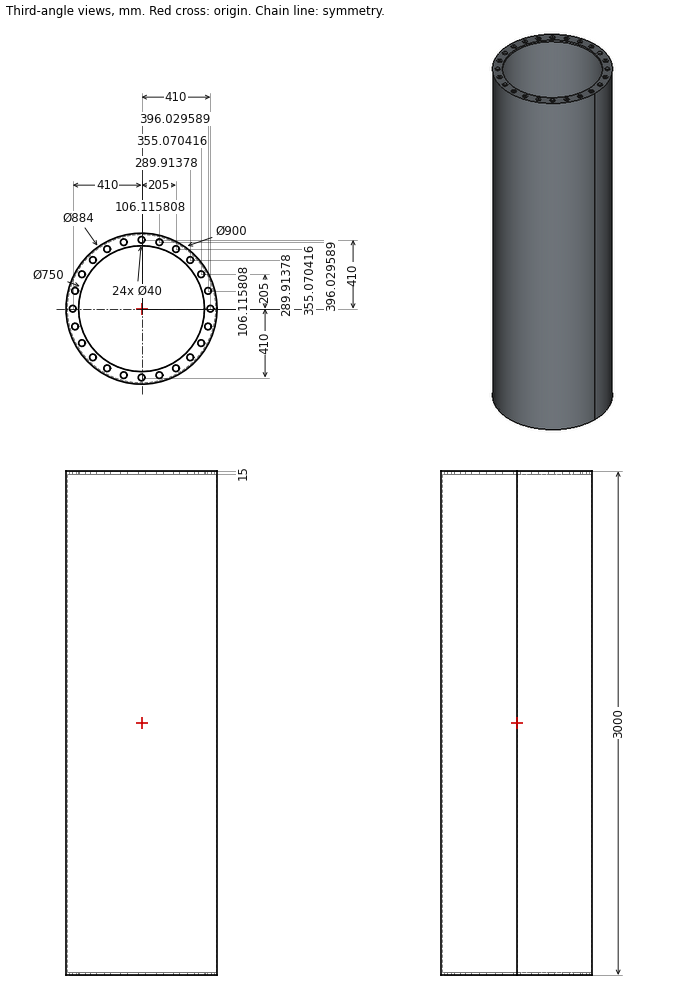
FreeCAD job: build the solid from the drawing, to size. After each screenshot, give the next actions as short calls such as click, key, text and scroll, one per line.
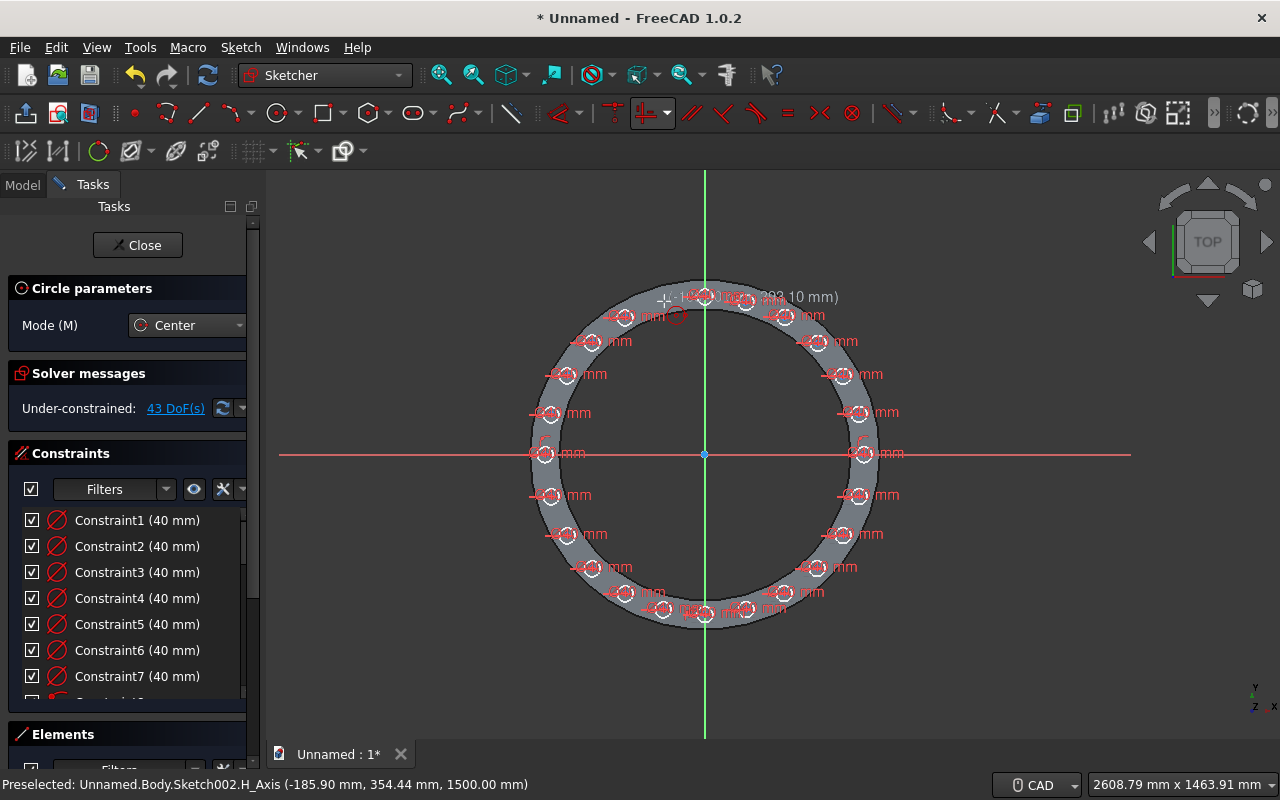
click(664, 301)
move(669, 295)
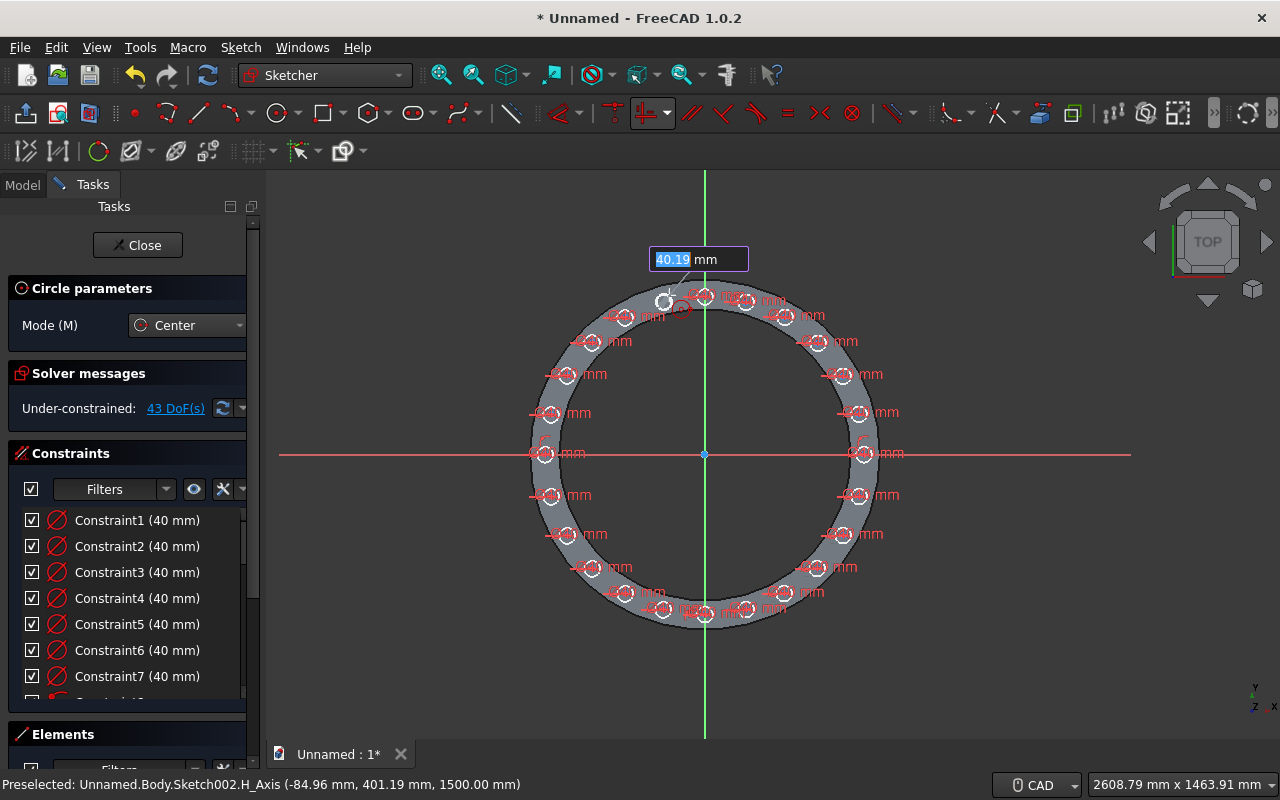
text(40)
key(Return)
key(Escape)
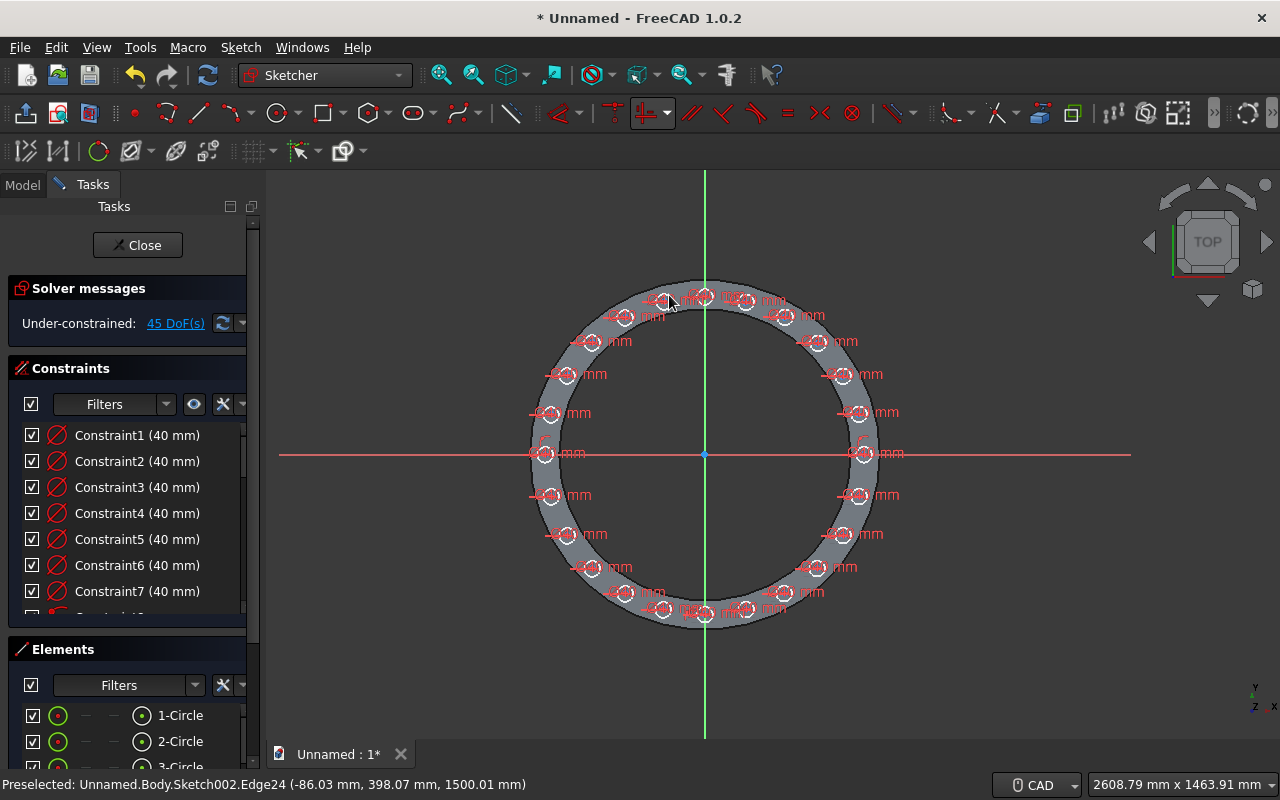
click(705, 297)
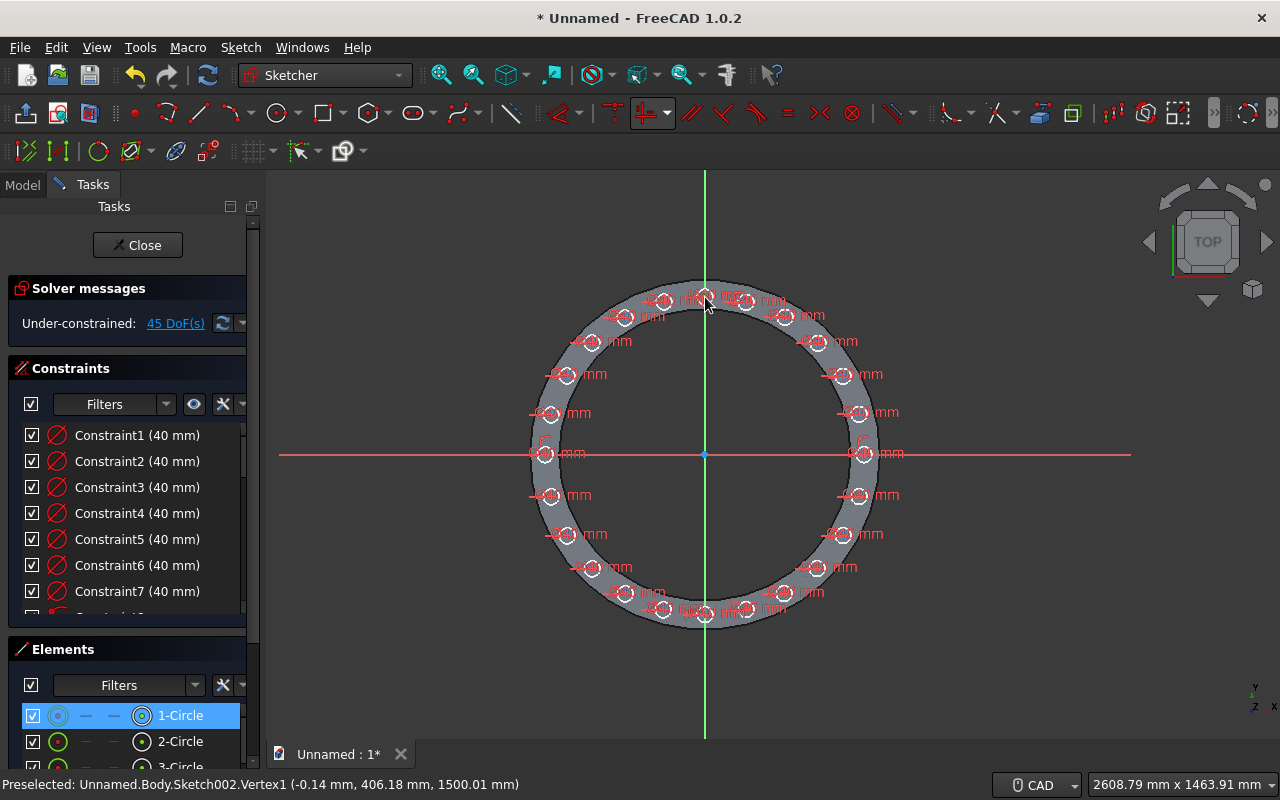
click(705, 674)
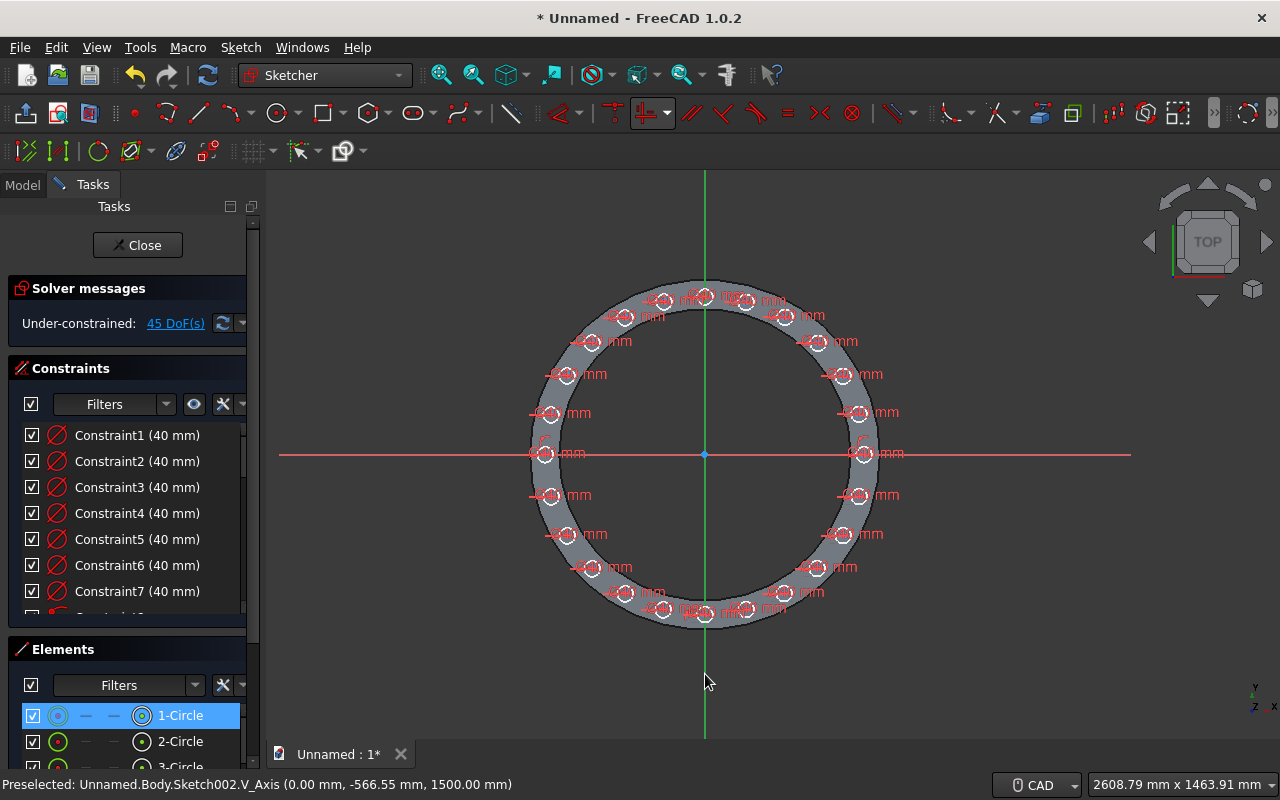
click(614, 114)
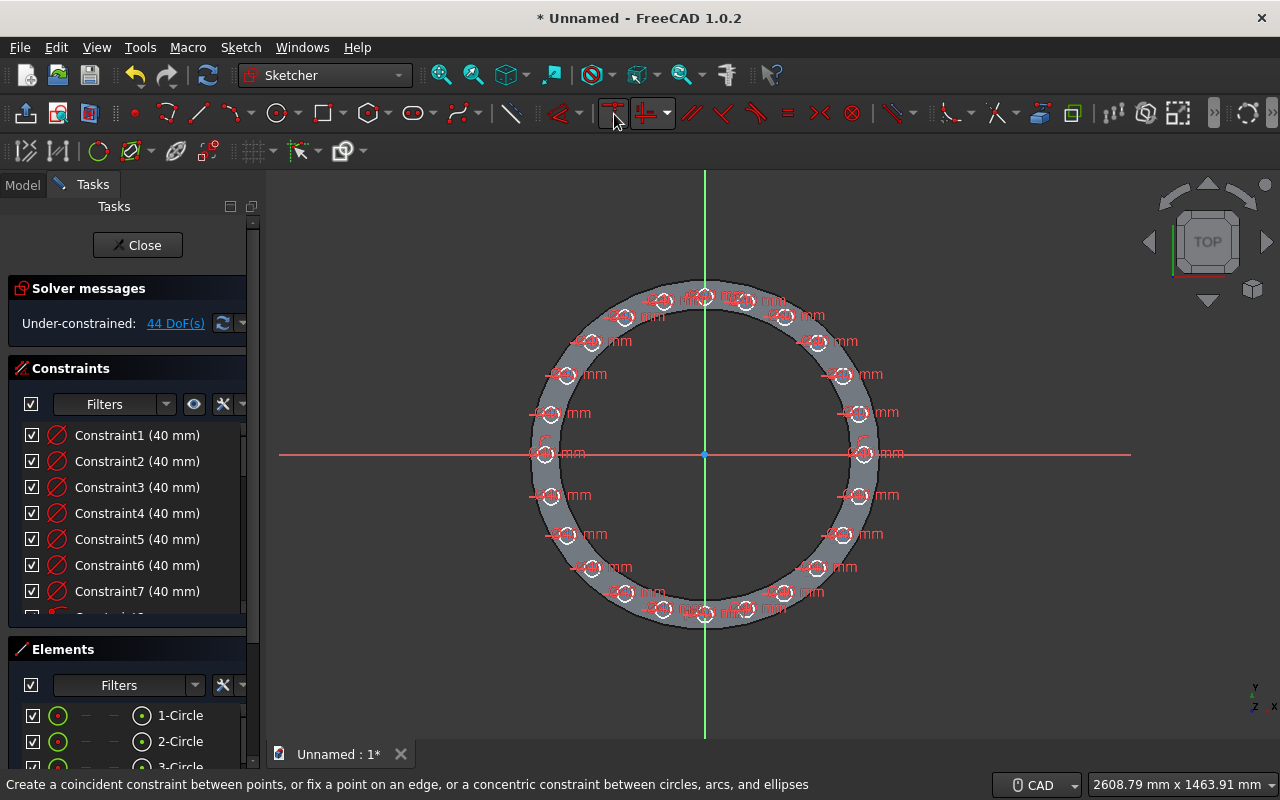
click(859, 414)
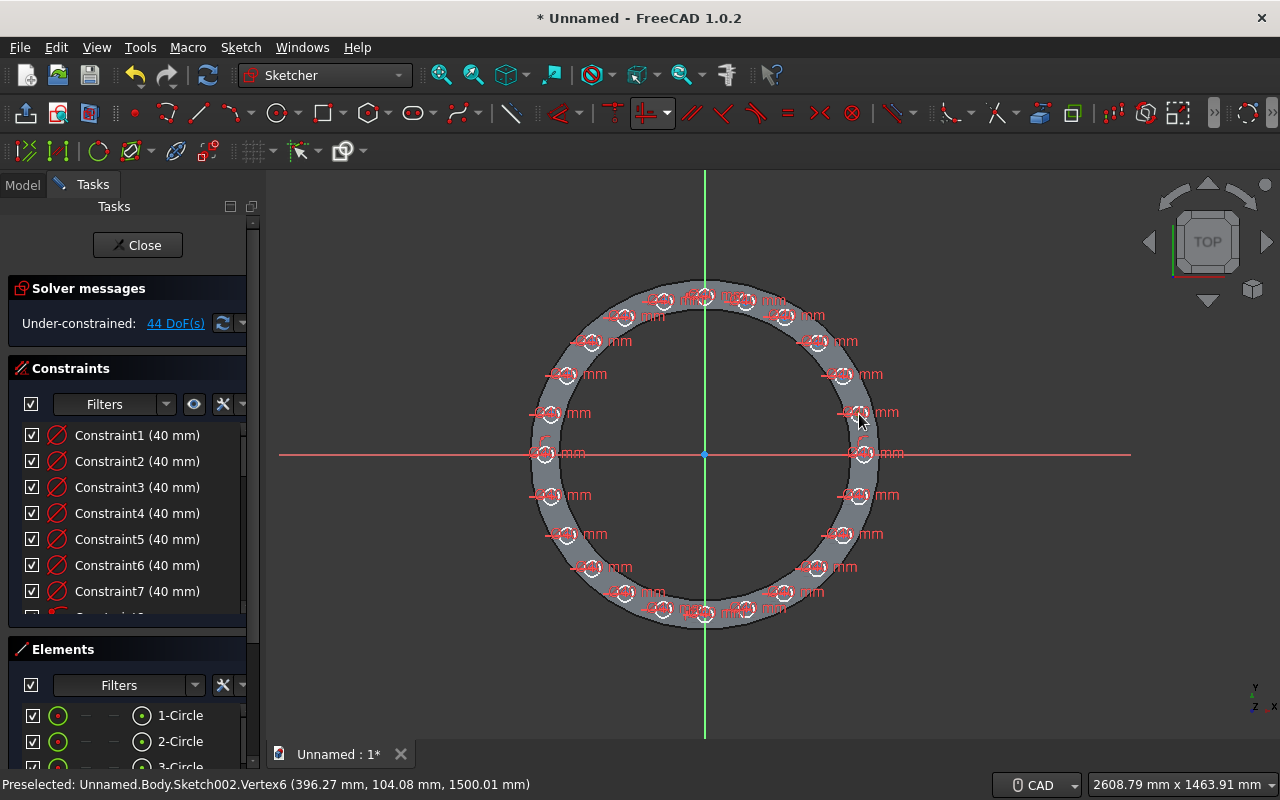
click(859, 497)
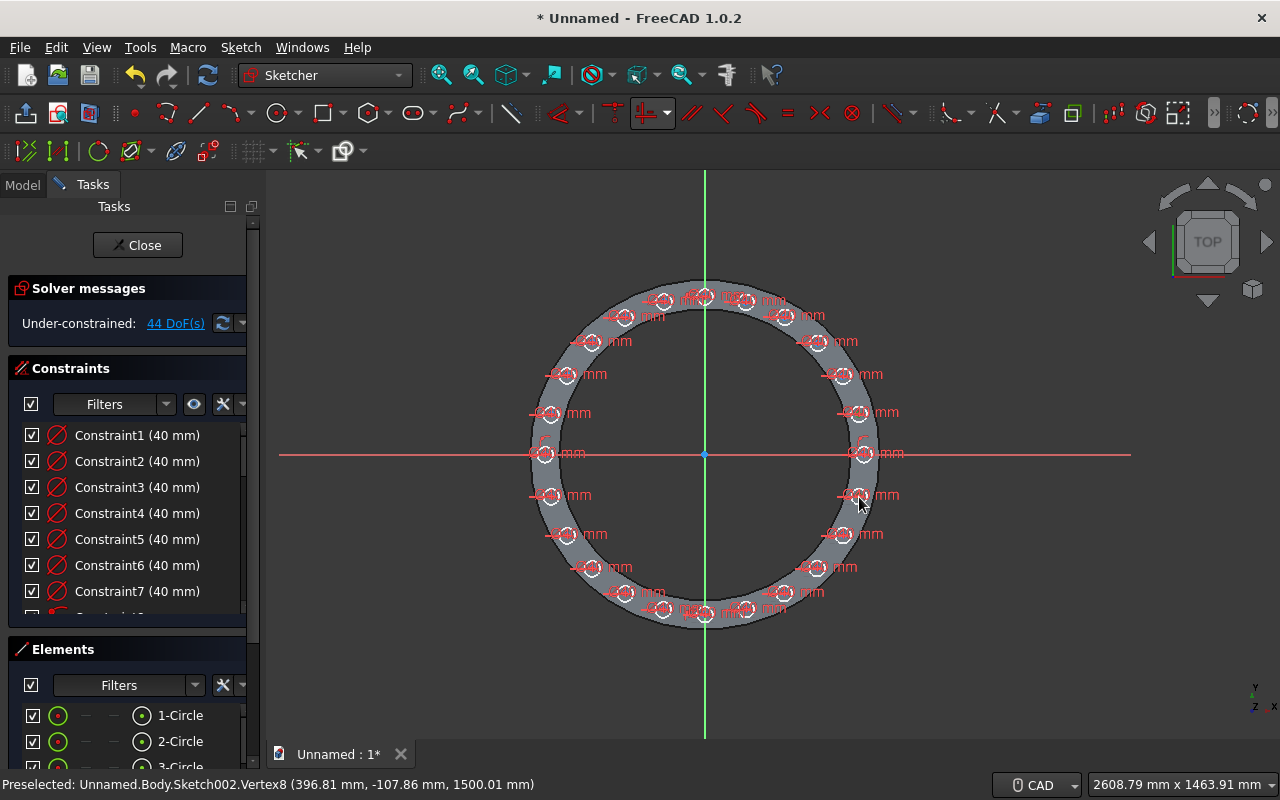
click(353, 455)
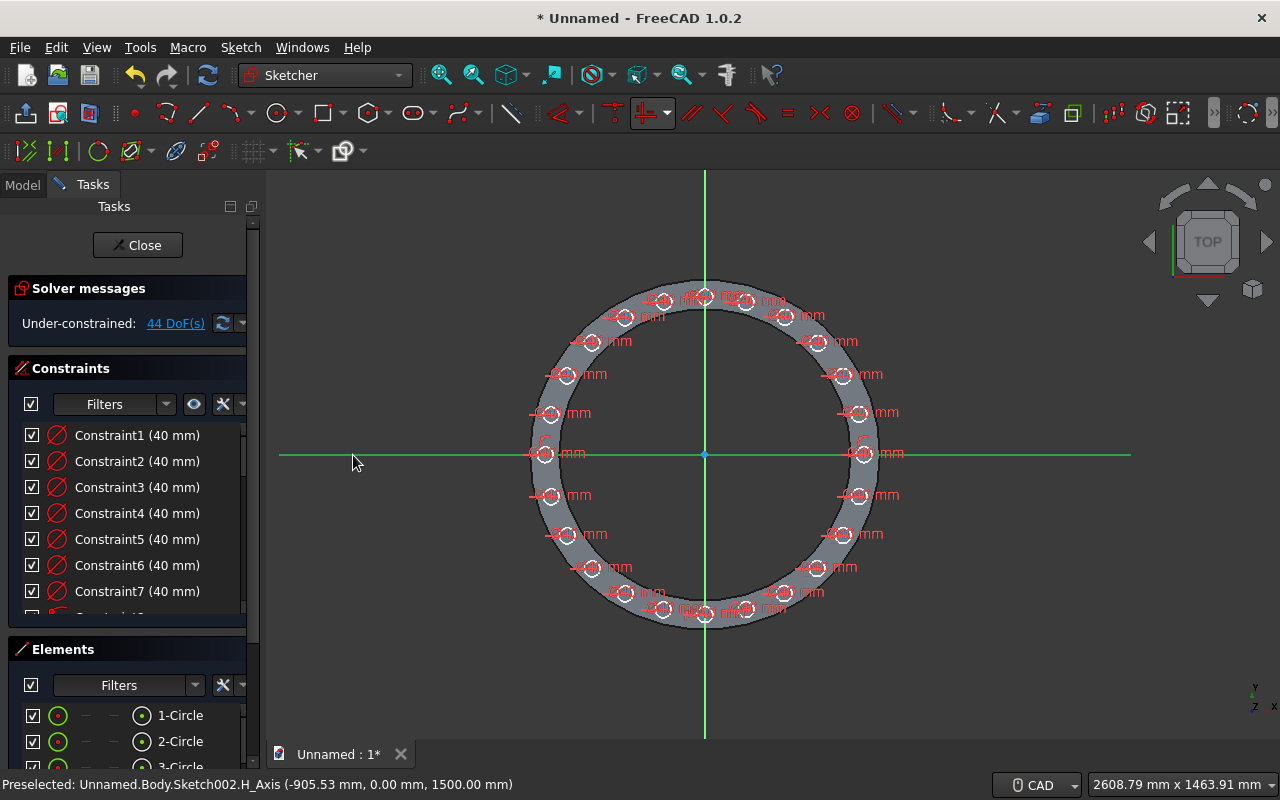
click(820, 114)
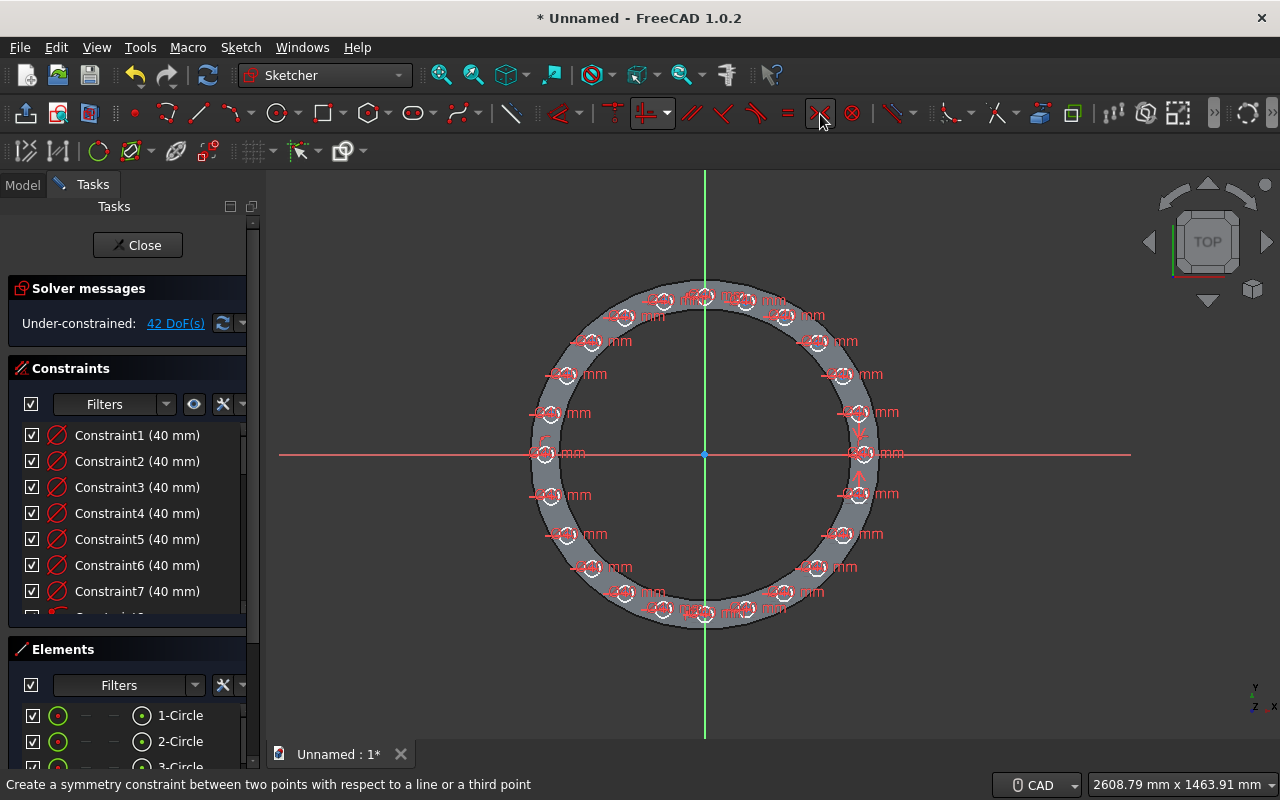
click(843, 376)